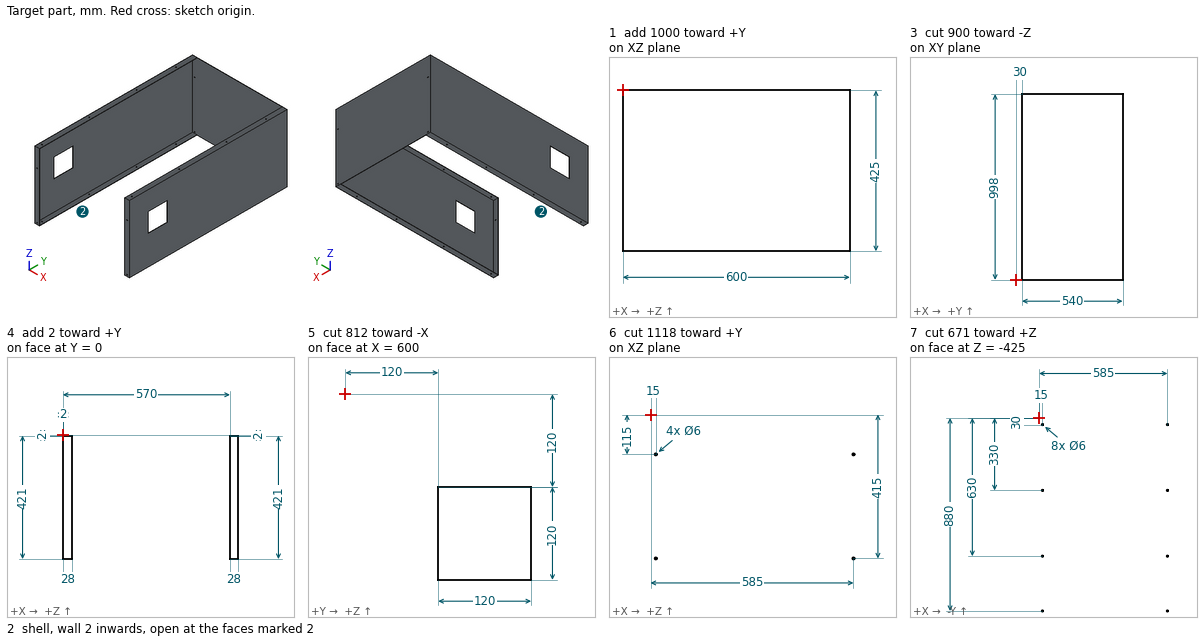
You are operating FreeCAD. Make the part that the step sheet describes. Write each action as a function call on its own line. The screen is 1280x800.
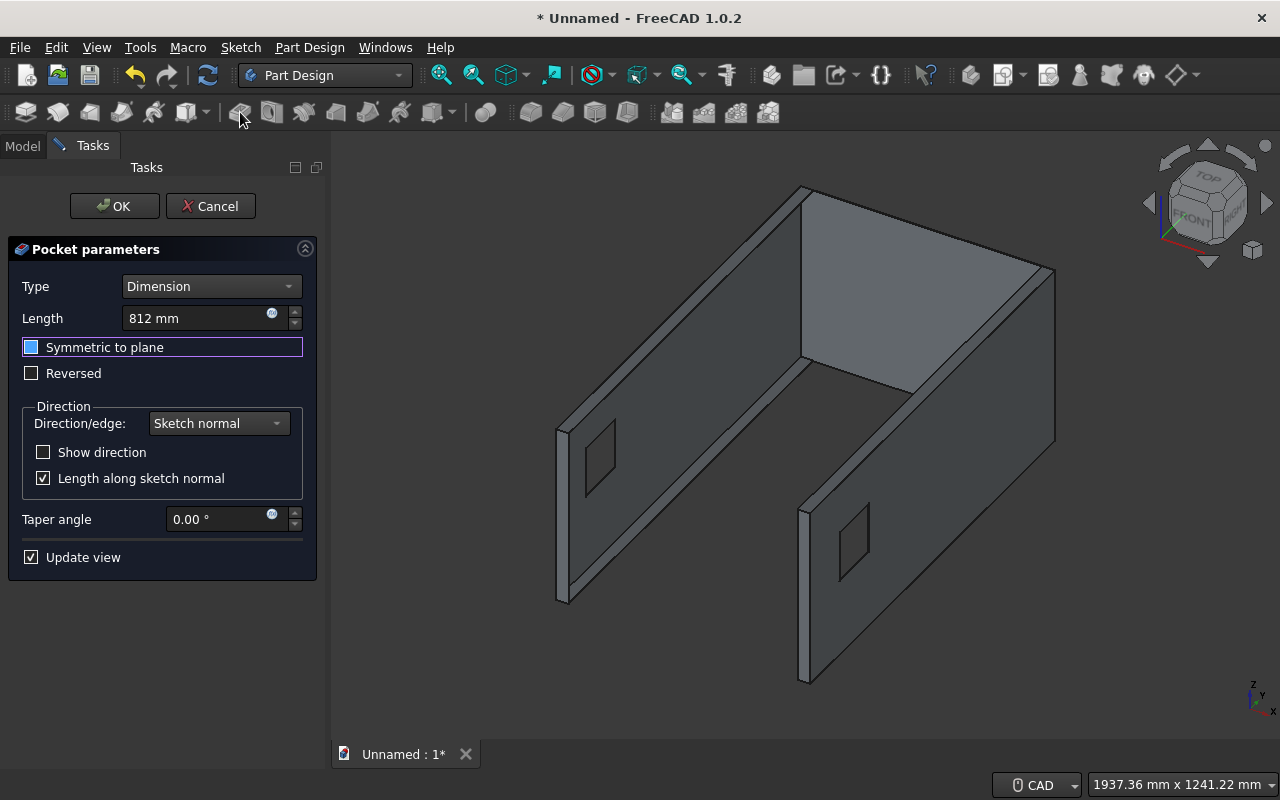
click(115, 206)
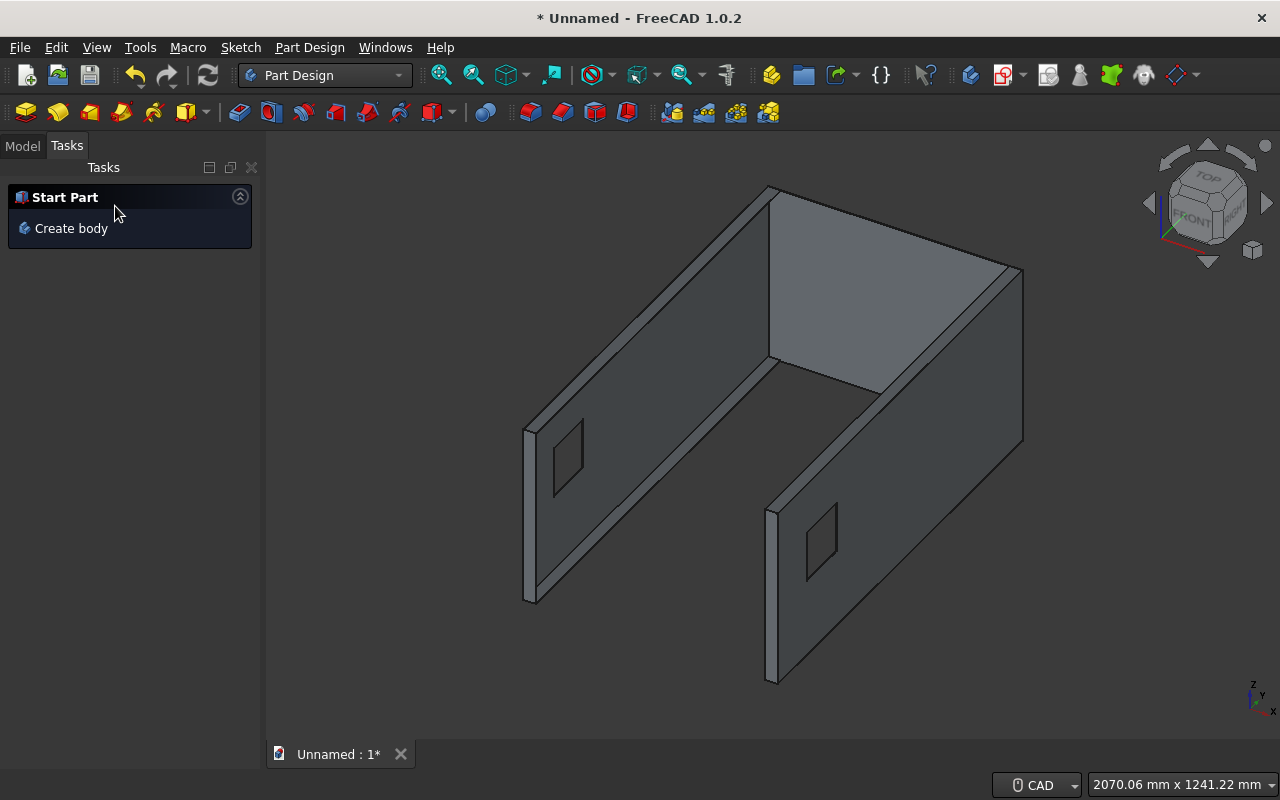
click(1004, 76)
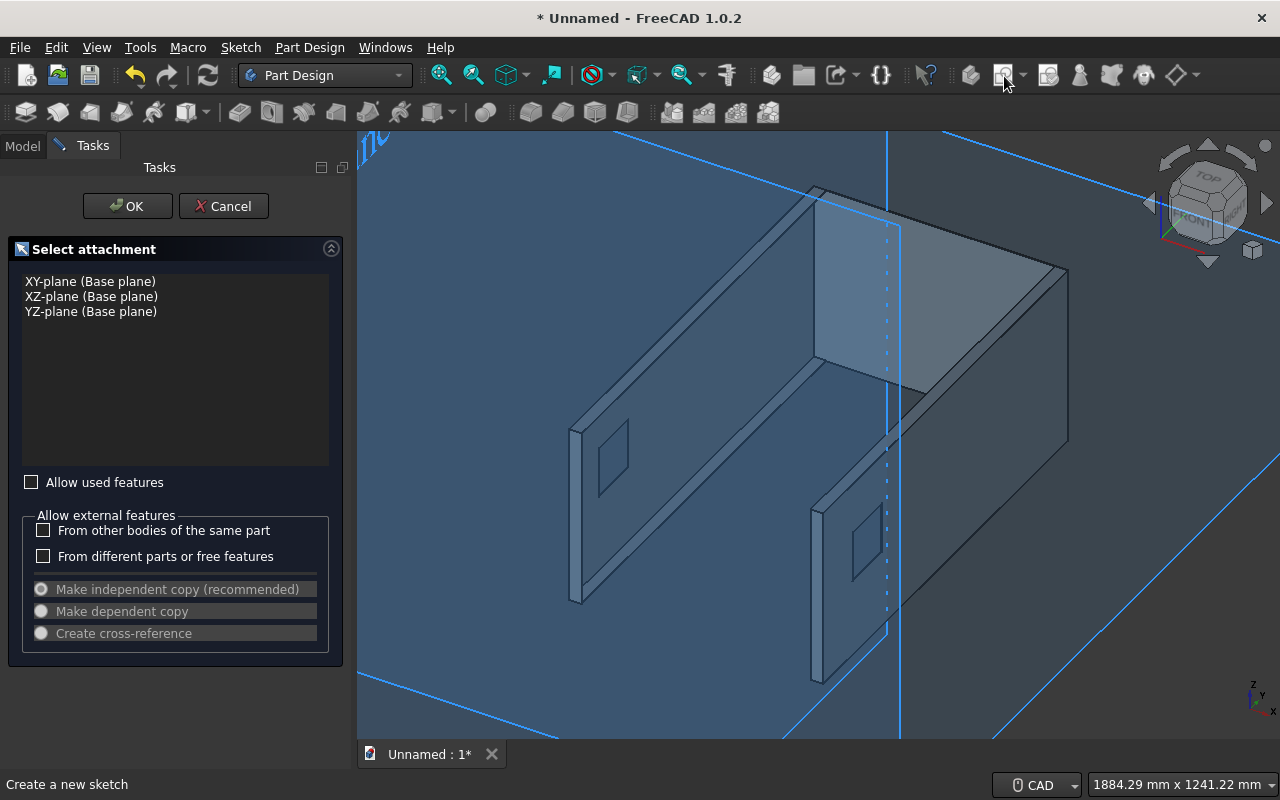
click(82, 296)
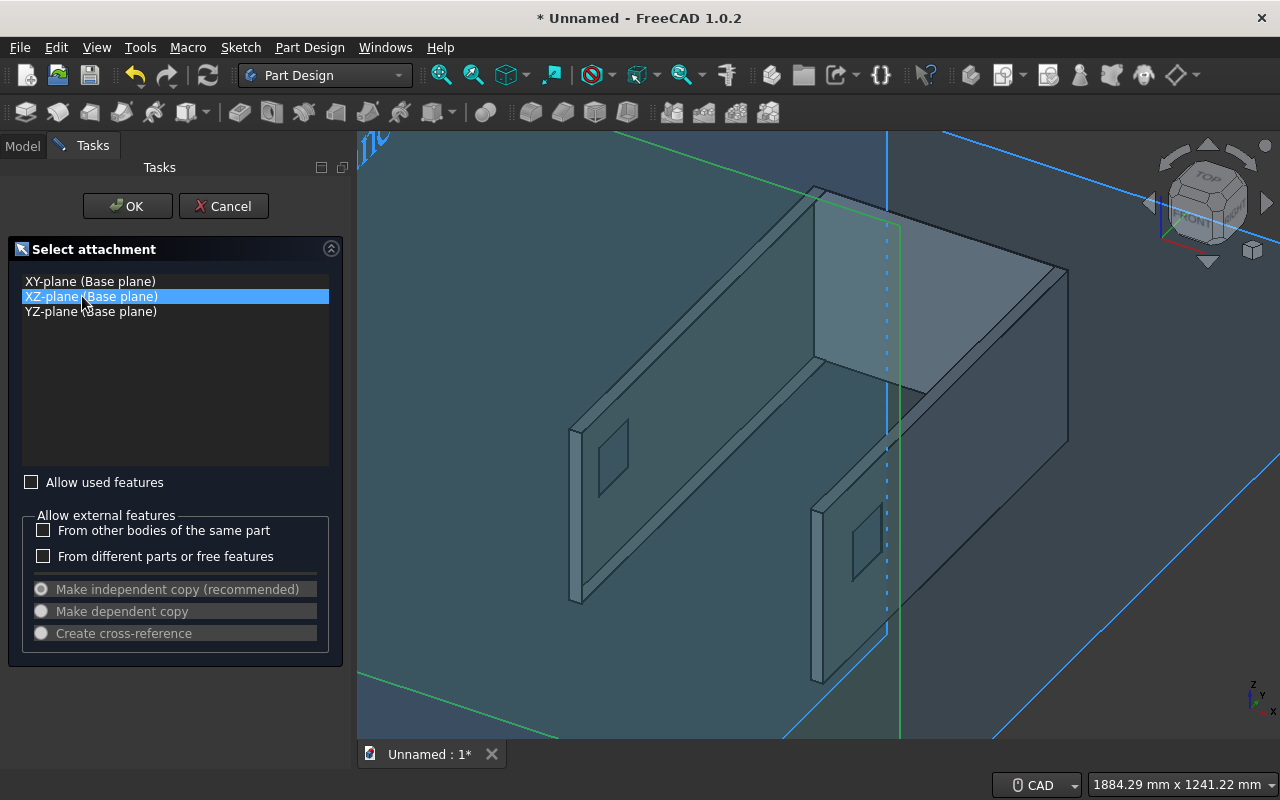
click(128, 206)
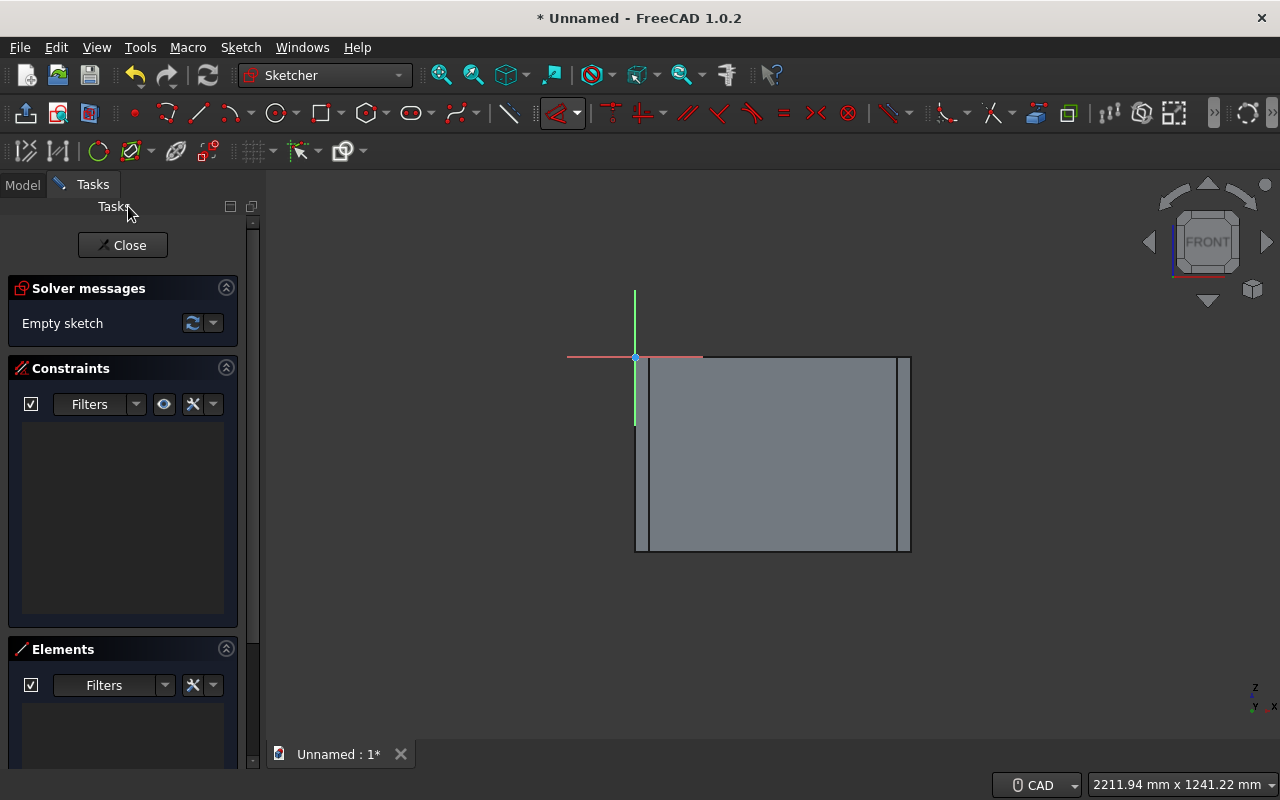
scroll(850, 451, up, 3)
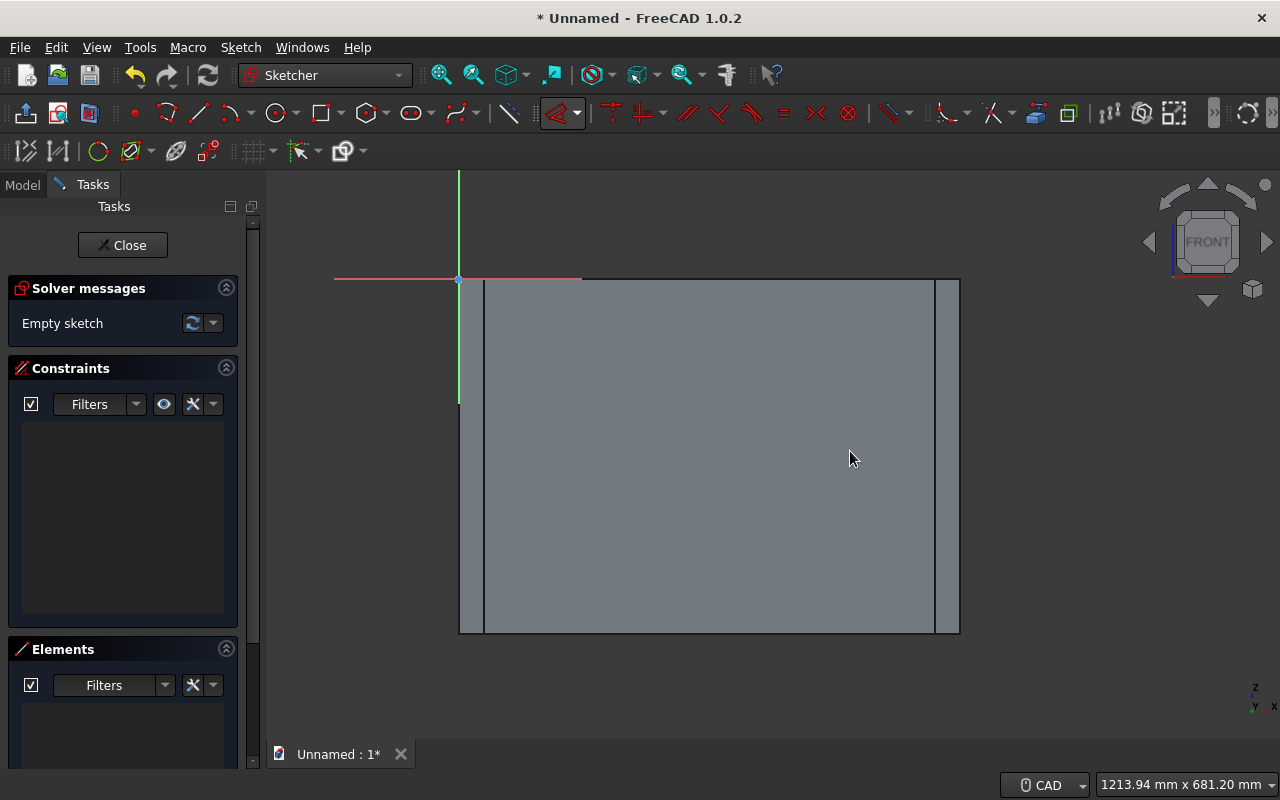
click(276, 114)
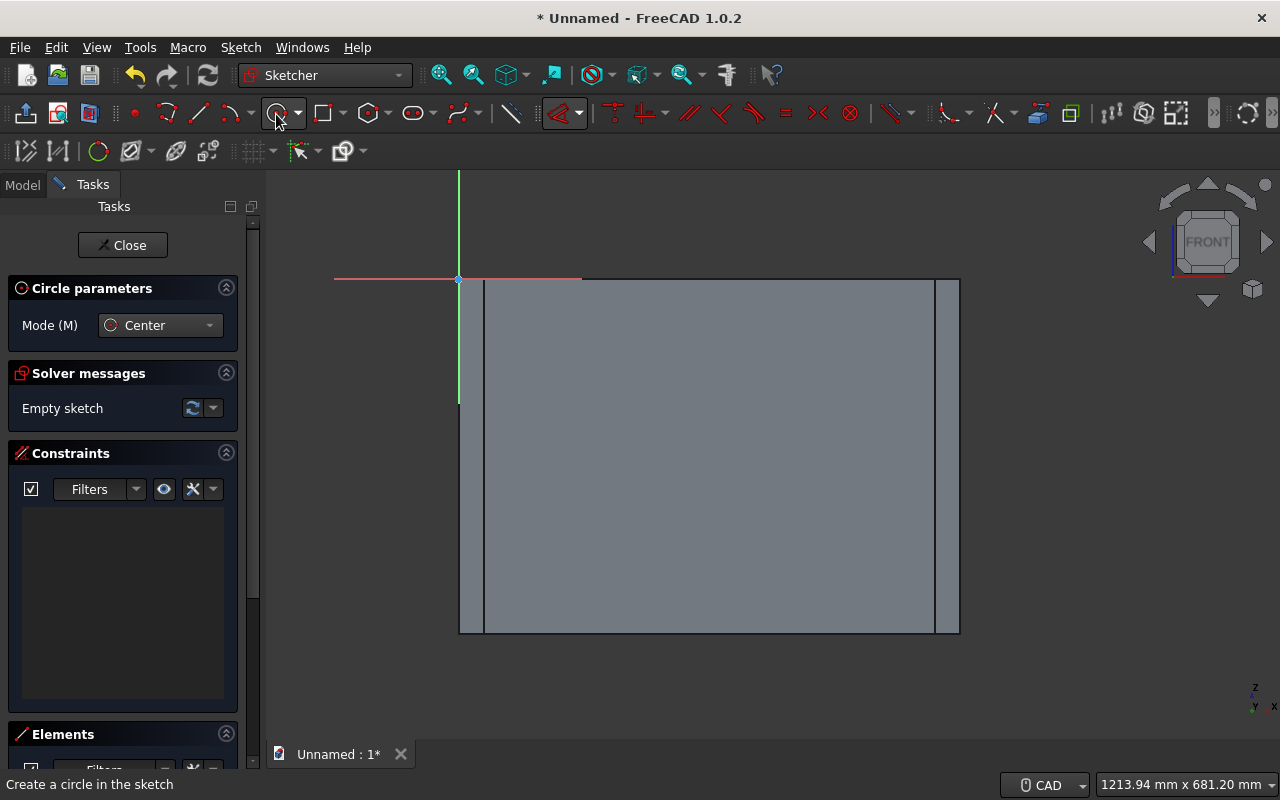
scroll(471, 376, up, 12)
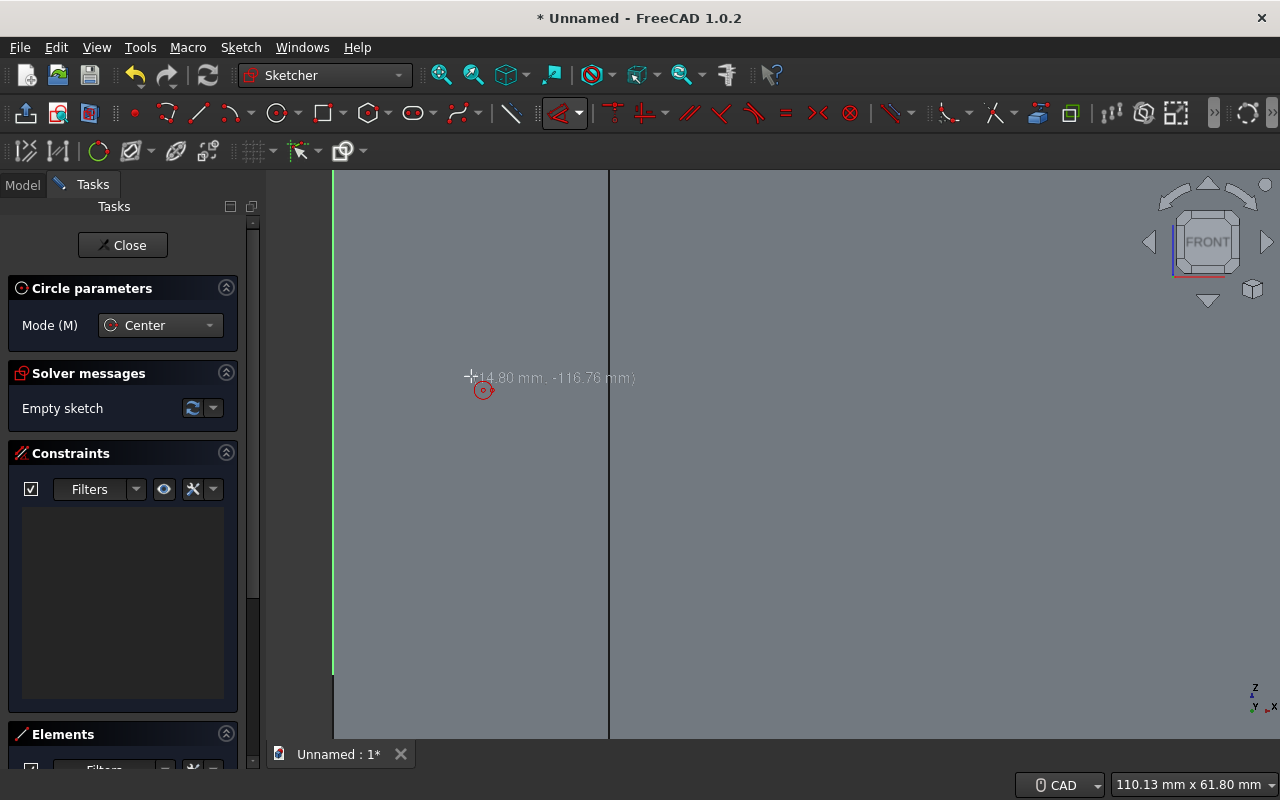
scroll(472, 377, down, 12)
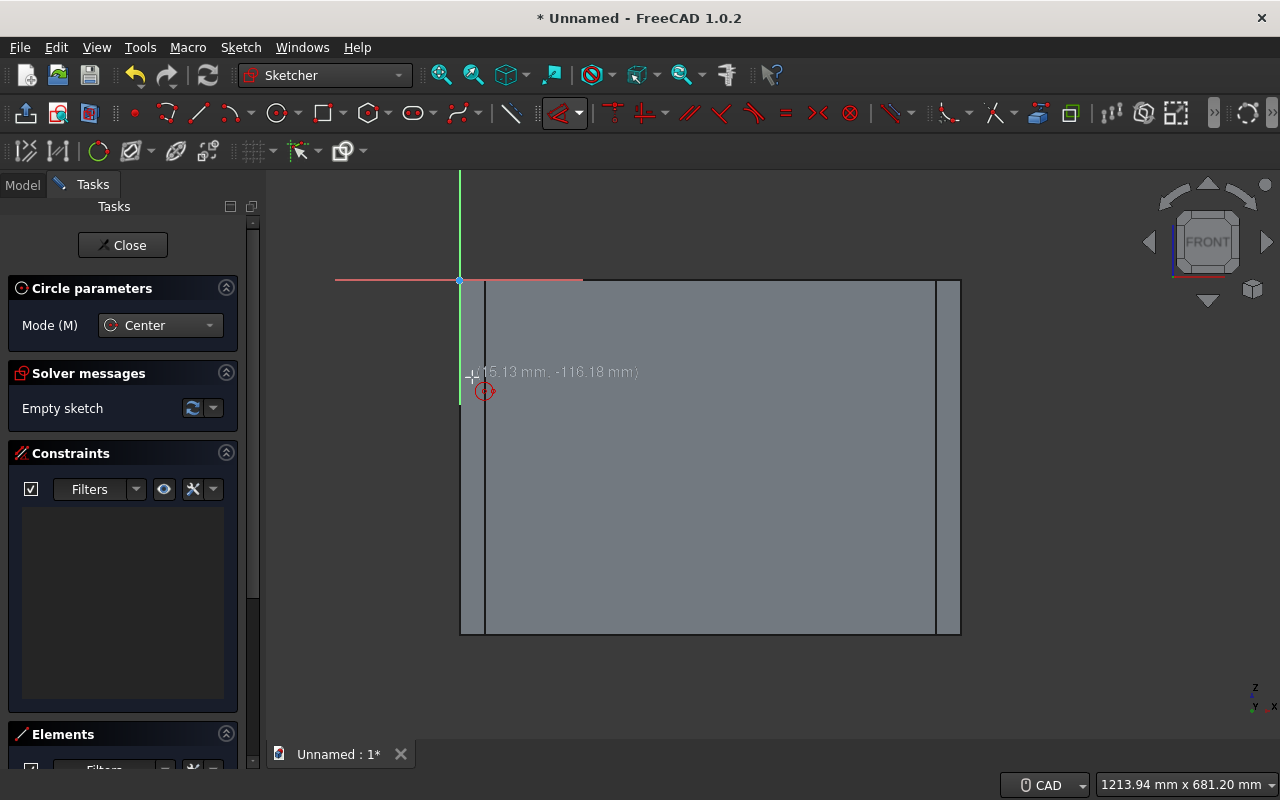
scroll(472, 376, up, 2)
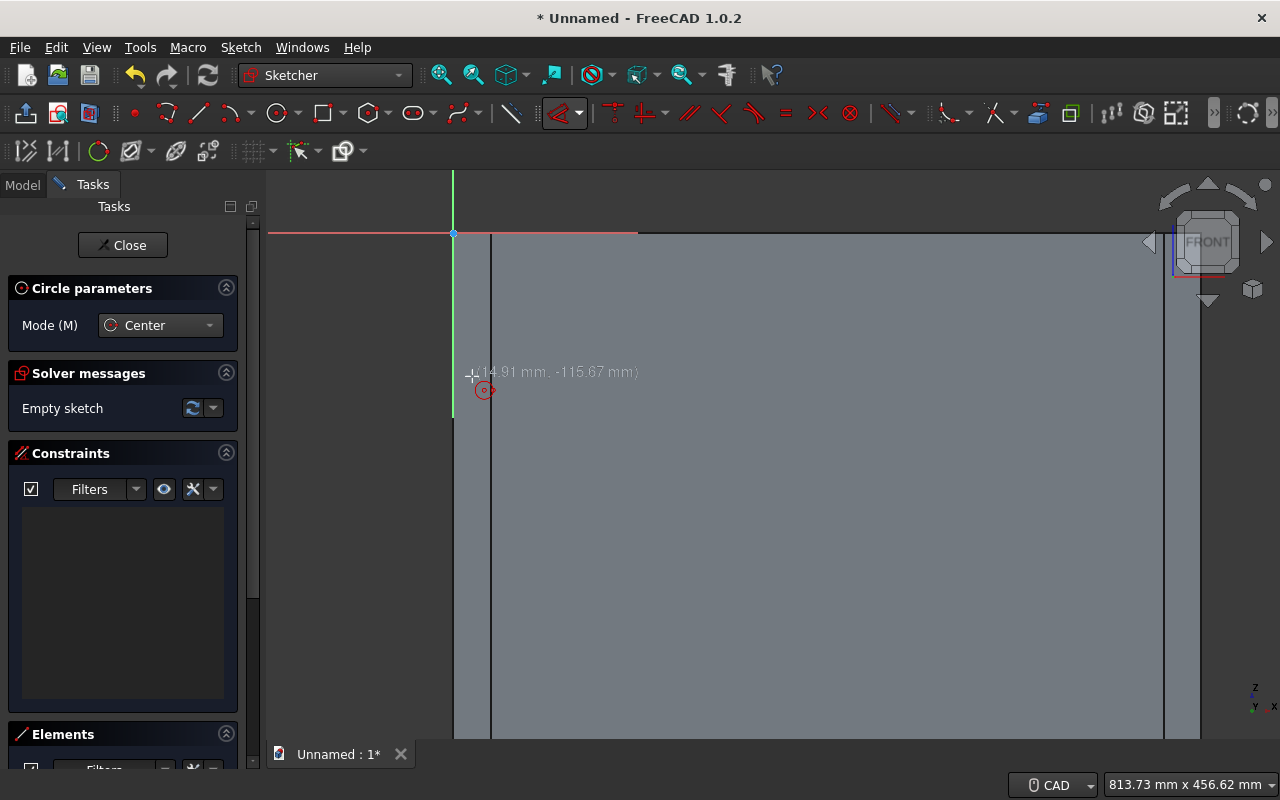
click(472, 376)
move(475, 374)